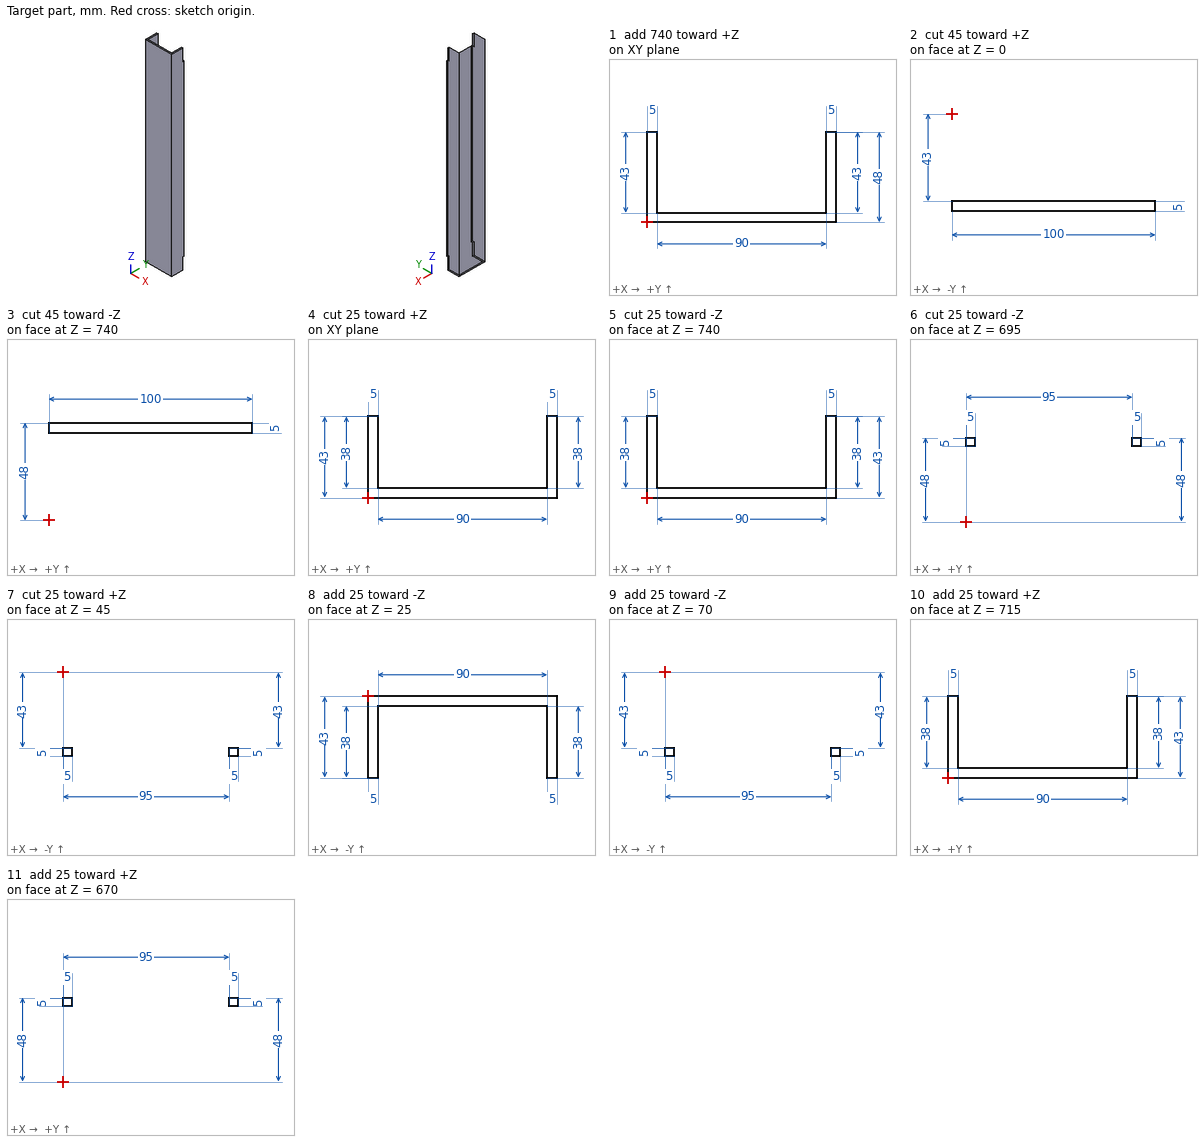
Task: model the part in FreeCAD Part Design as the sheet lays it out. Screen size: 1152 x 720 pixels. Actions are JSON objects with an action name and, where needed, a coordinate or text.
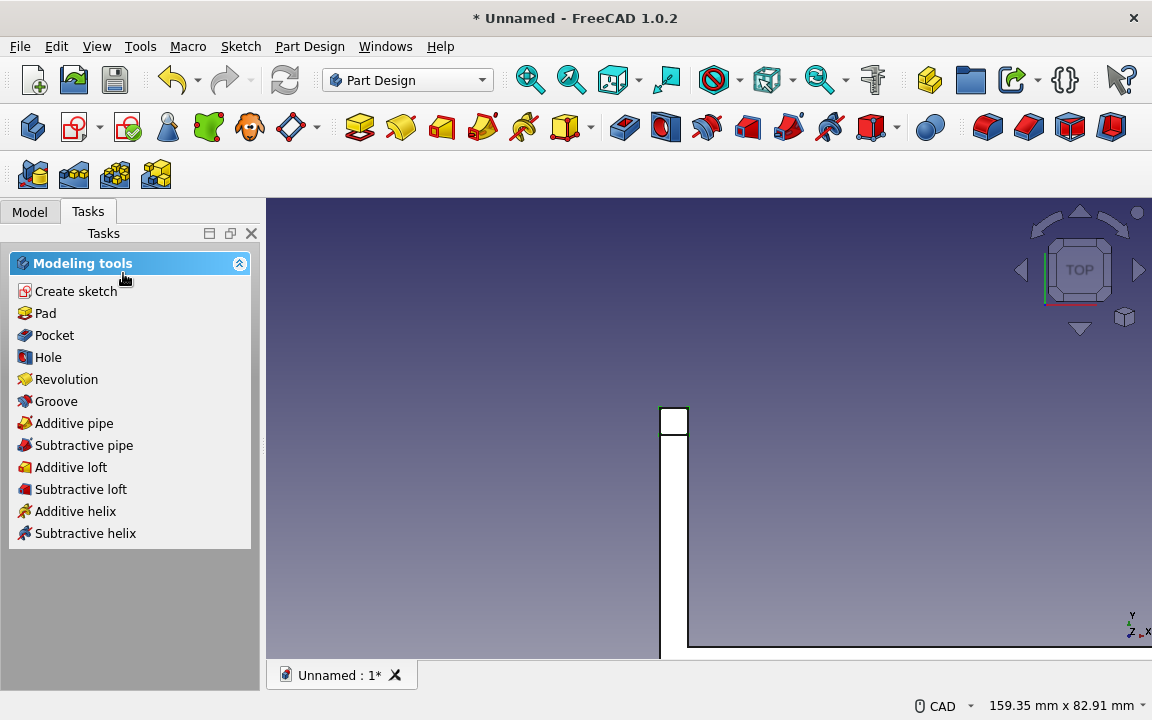
{"action": "left_click", "coordinate": [360, 128]}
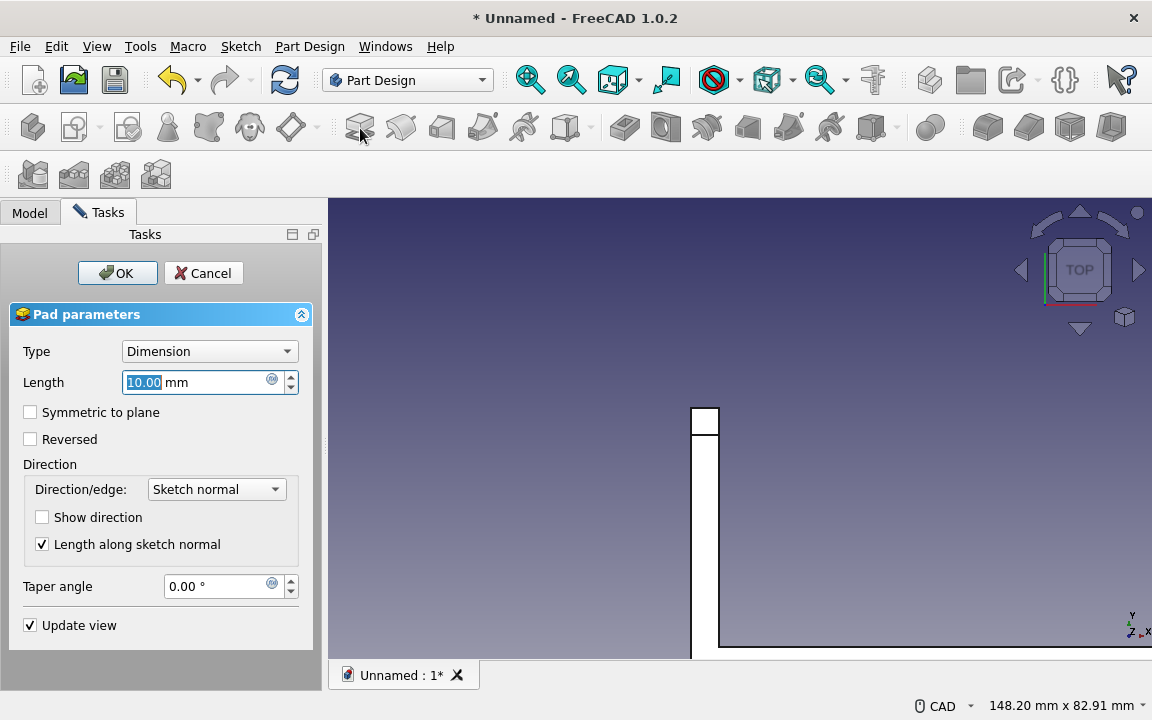
{"action": "type", "text": "25"}
{"action": "key", "text": "Tab"}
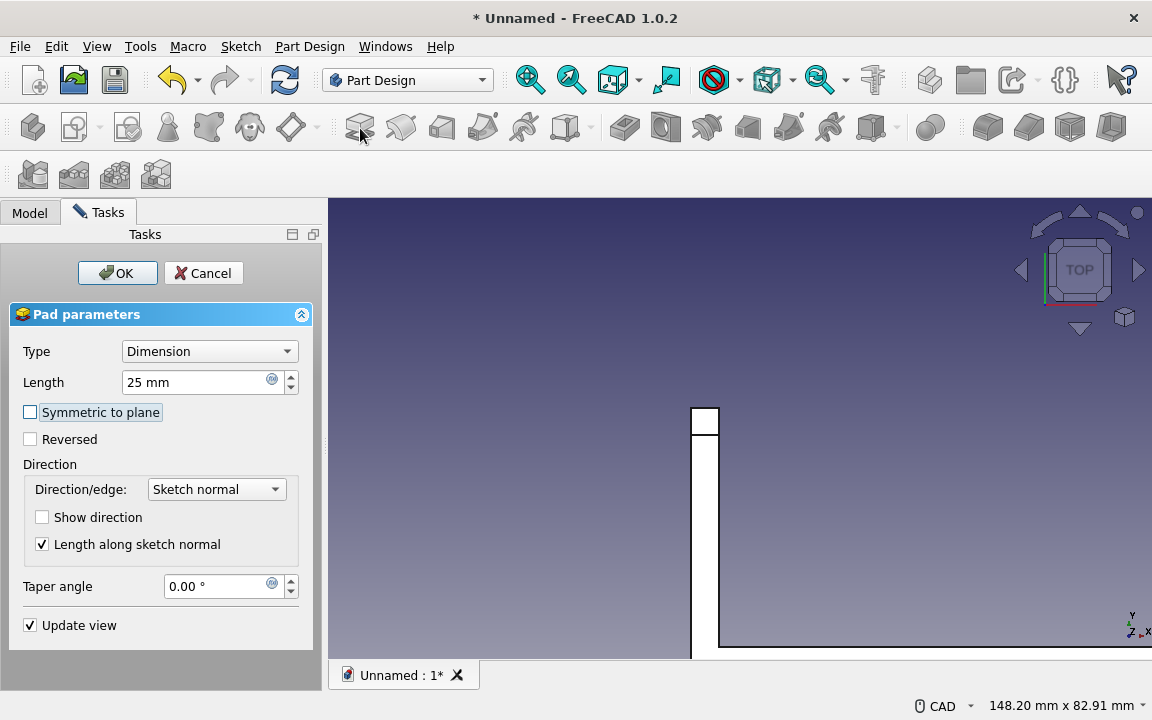
{"action": "left_click", "coordinate": [118, 273]}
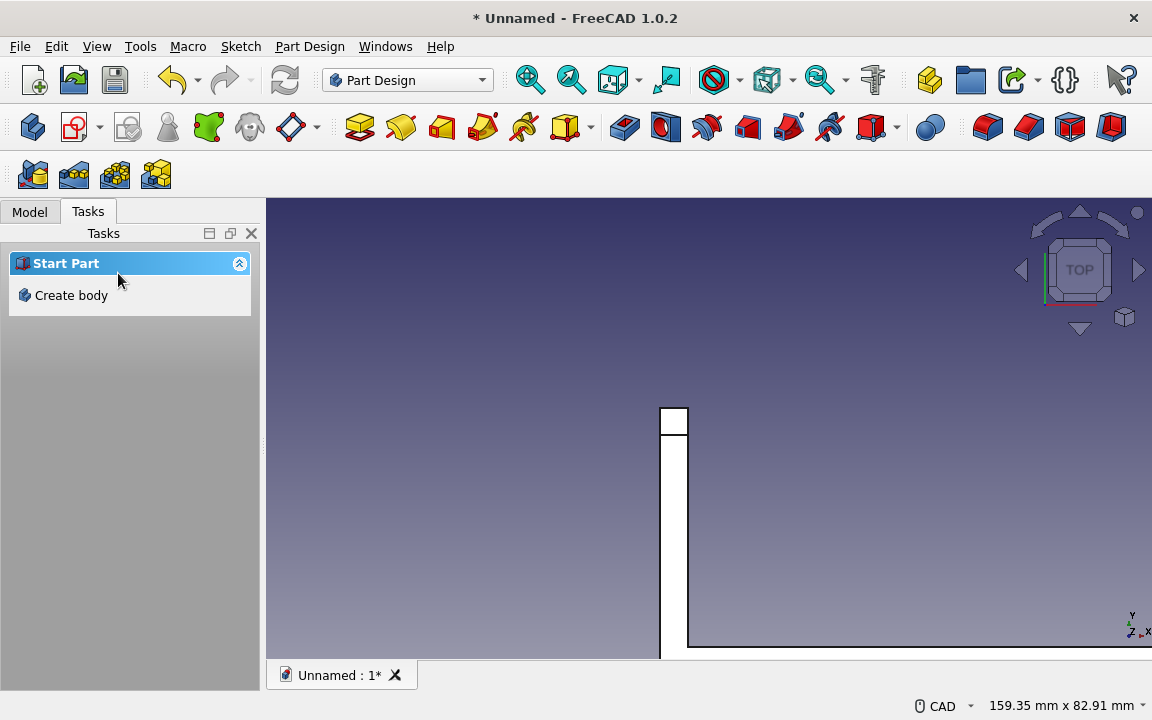
{"action": "key", "text": "0"}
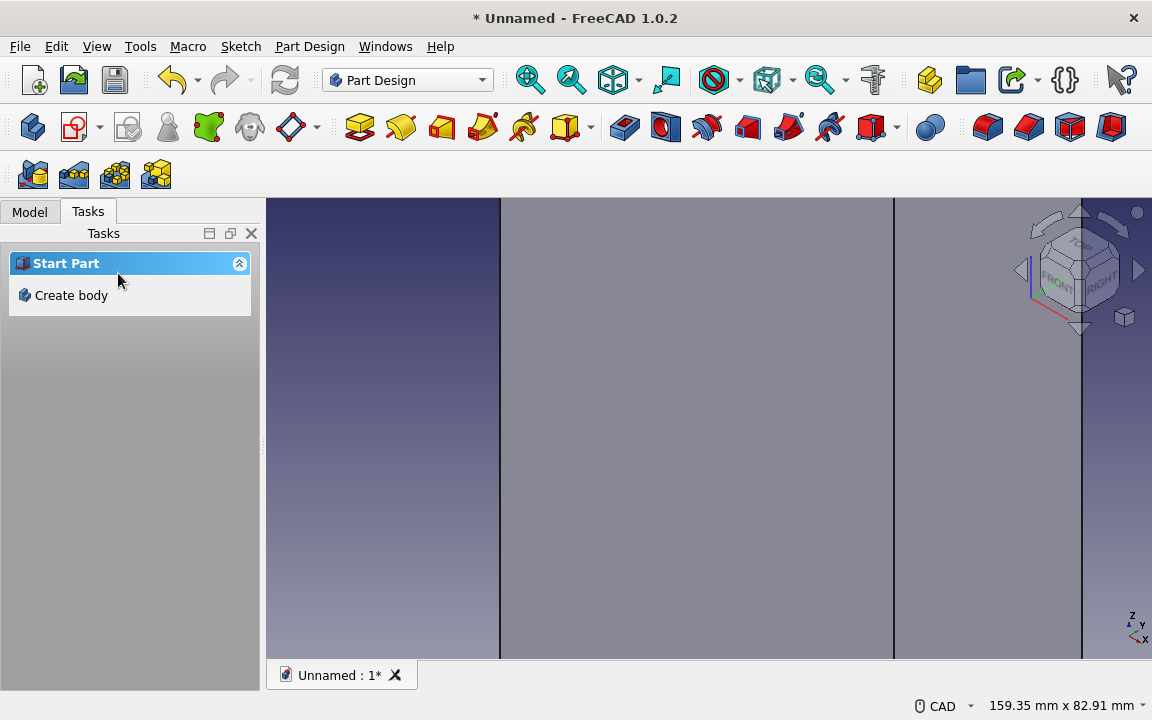
{"action": "key", "text": "v f"}